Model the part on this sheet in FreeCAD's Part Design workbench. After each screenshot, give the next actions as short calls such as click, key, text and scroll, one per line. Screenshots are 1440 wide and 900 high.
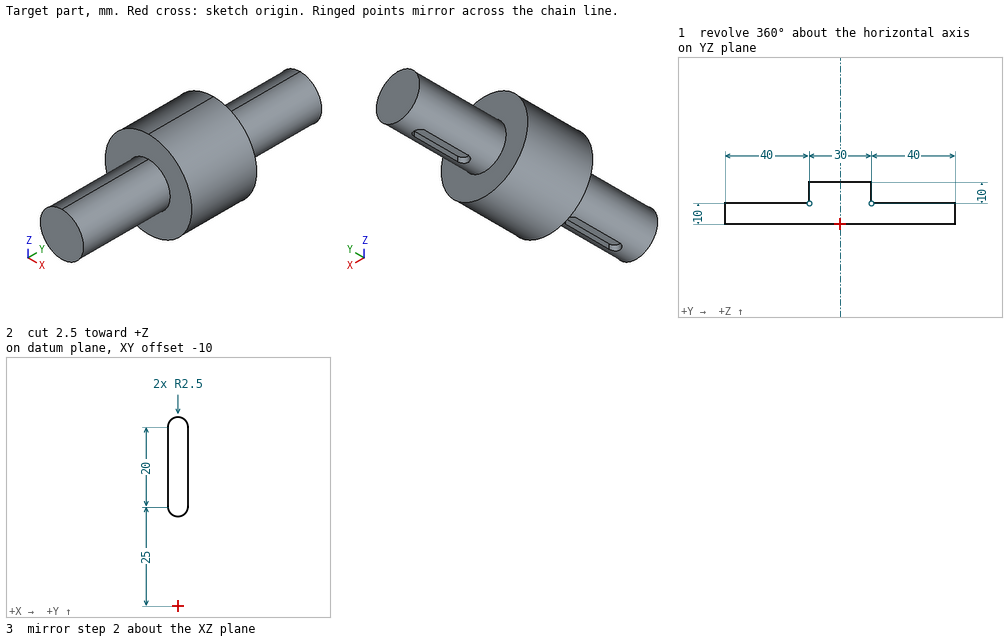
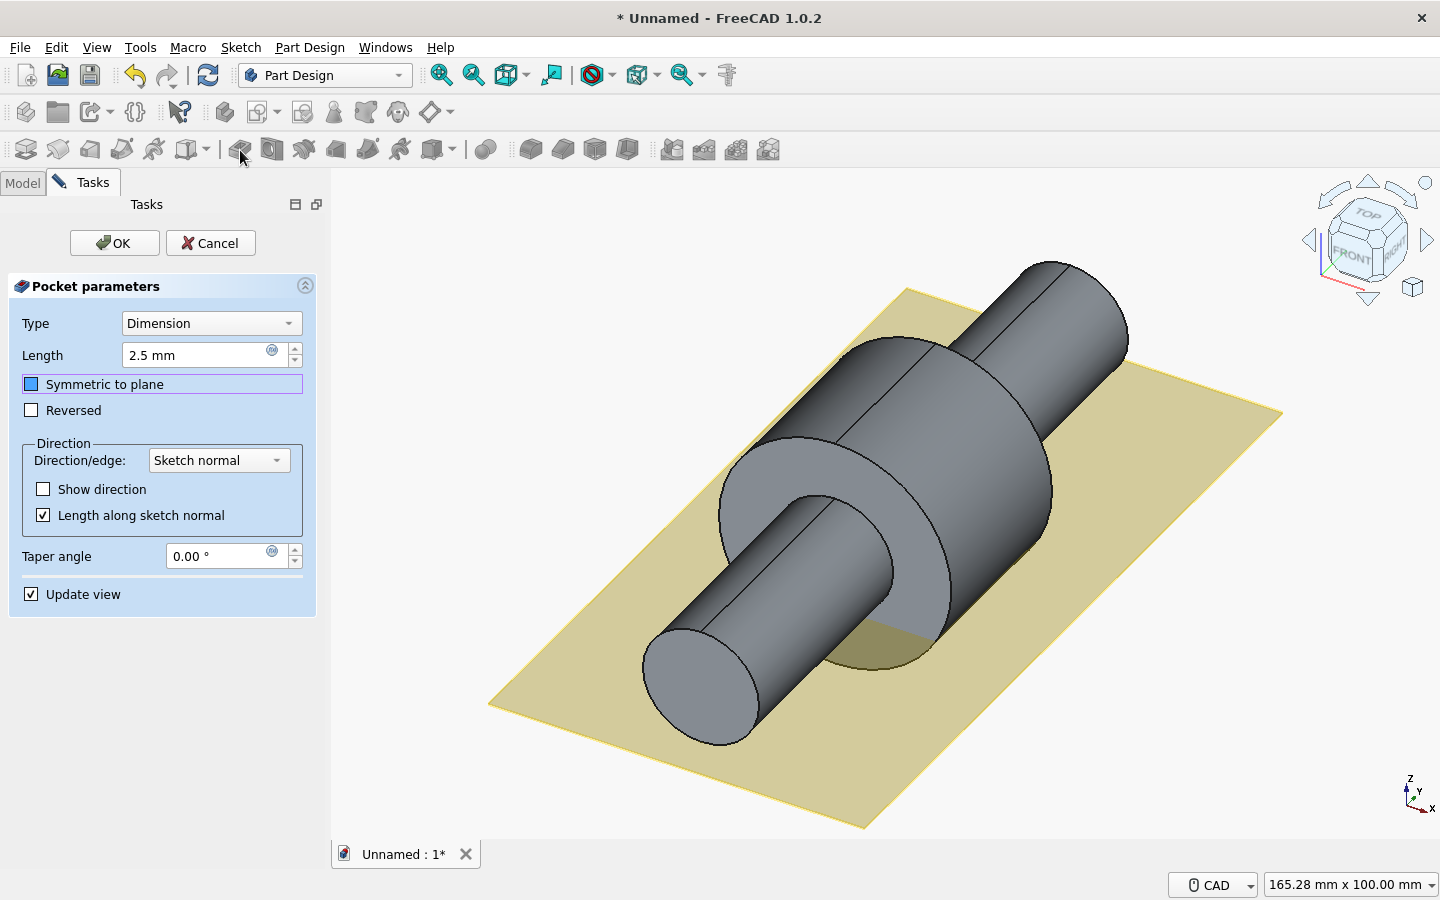
click(30, 410)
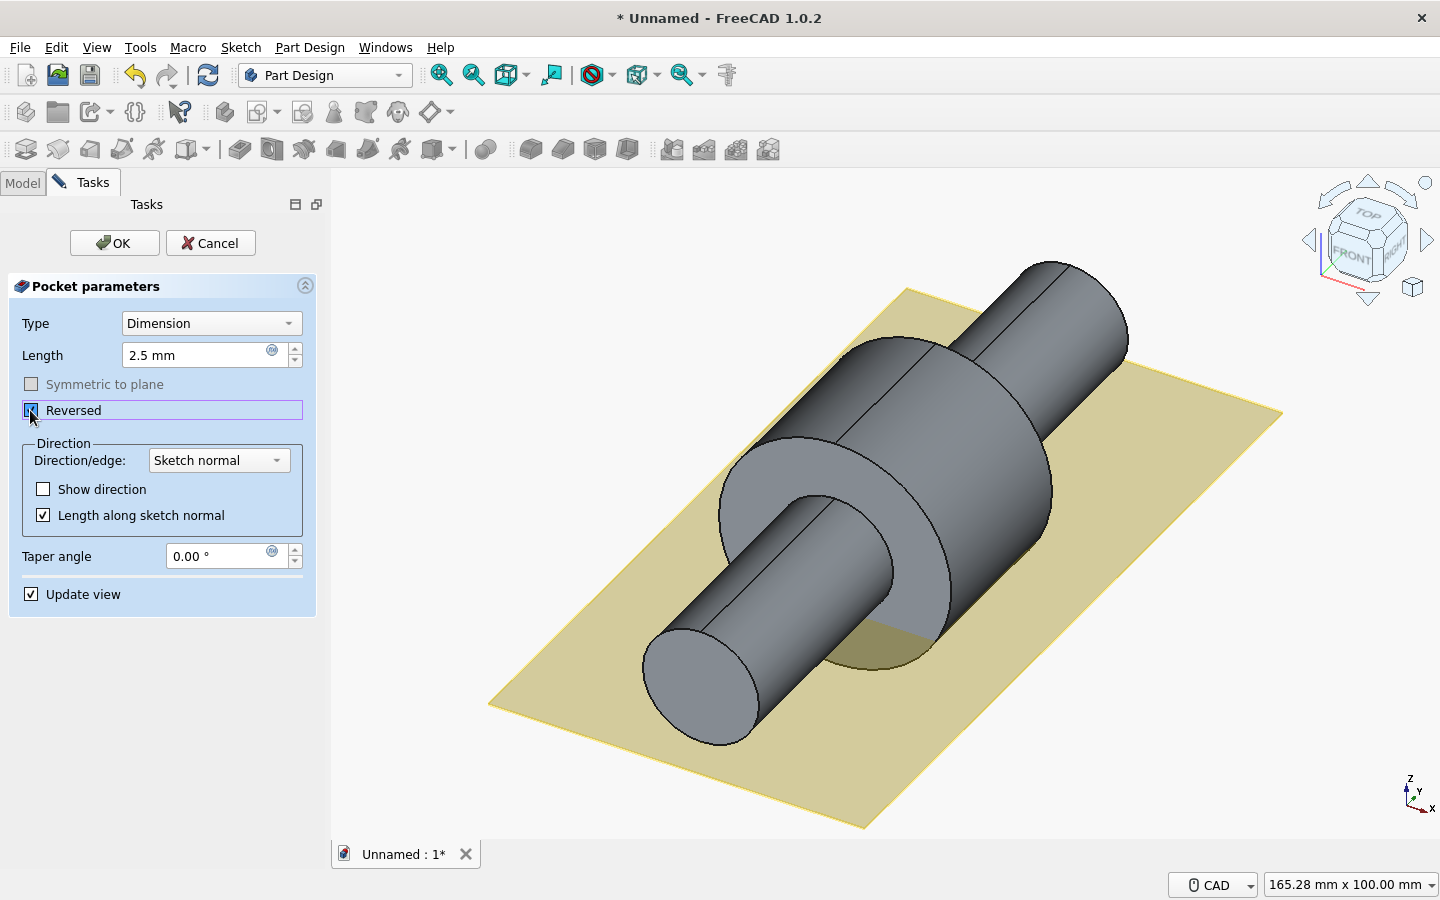
click(115, 243)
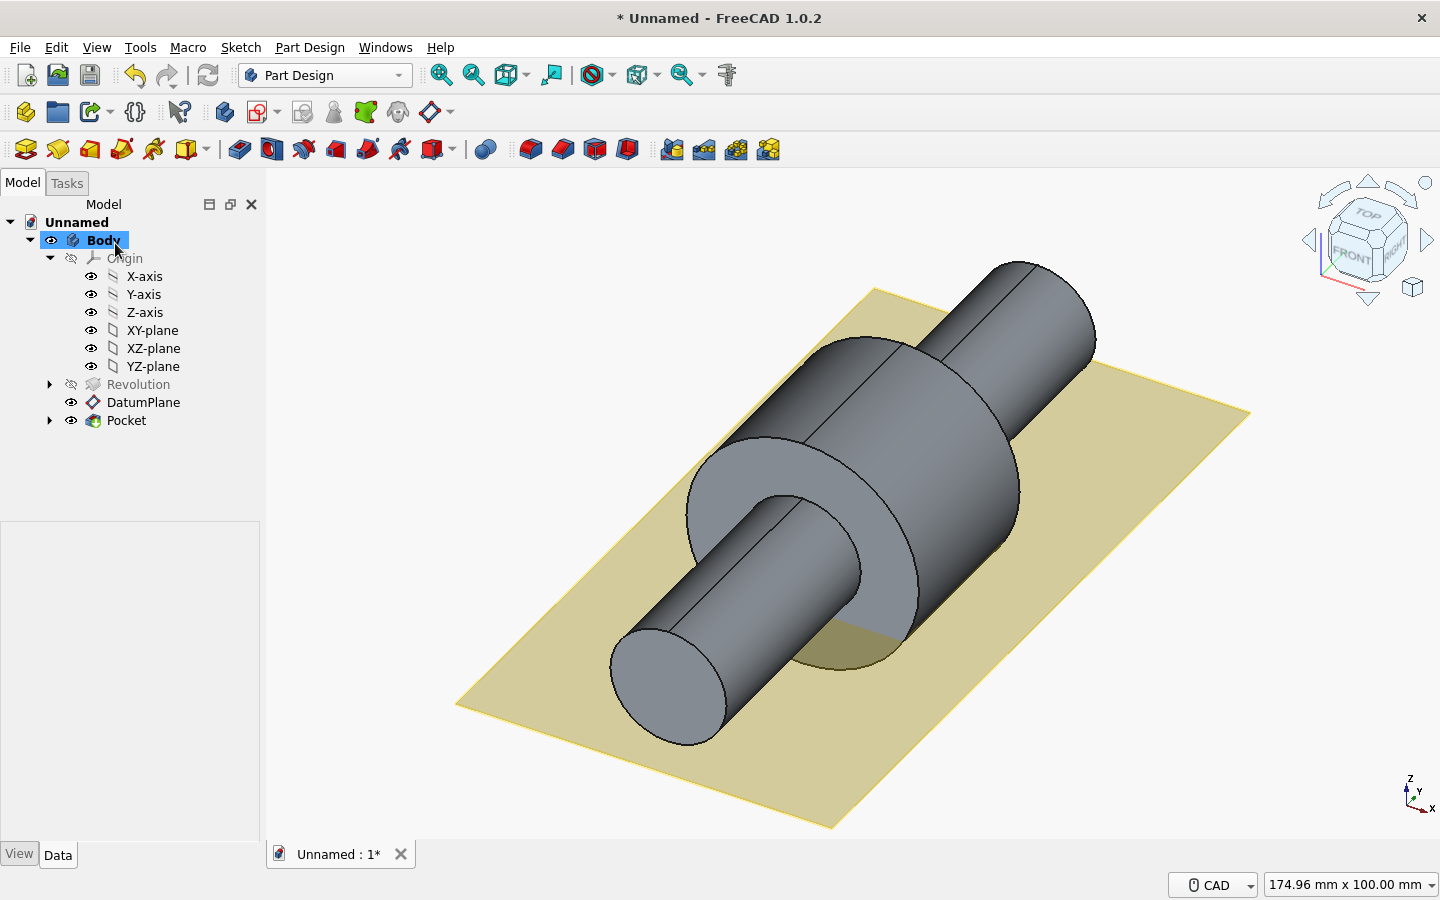
click(116, 402)
key(space)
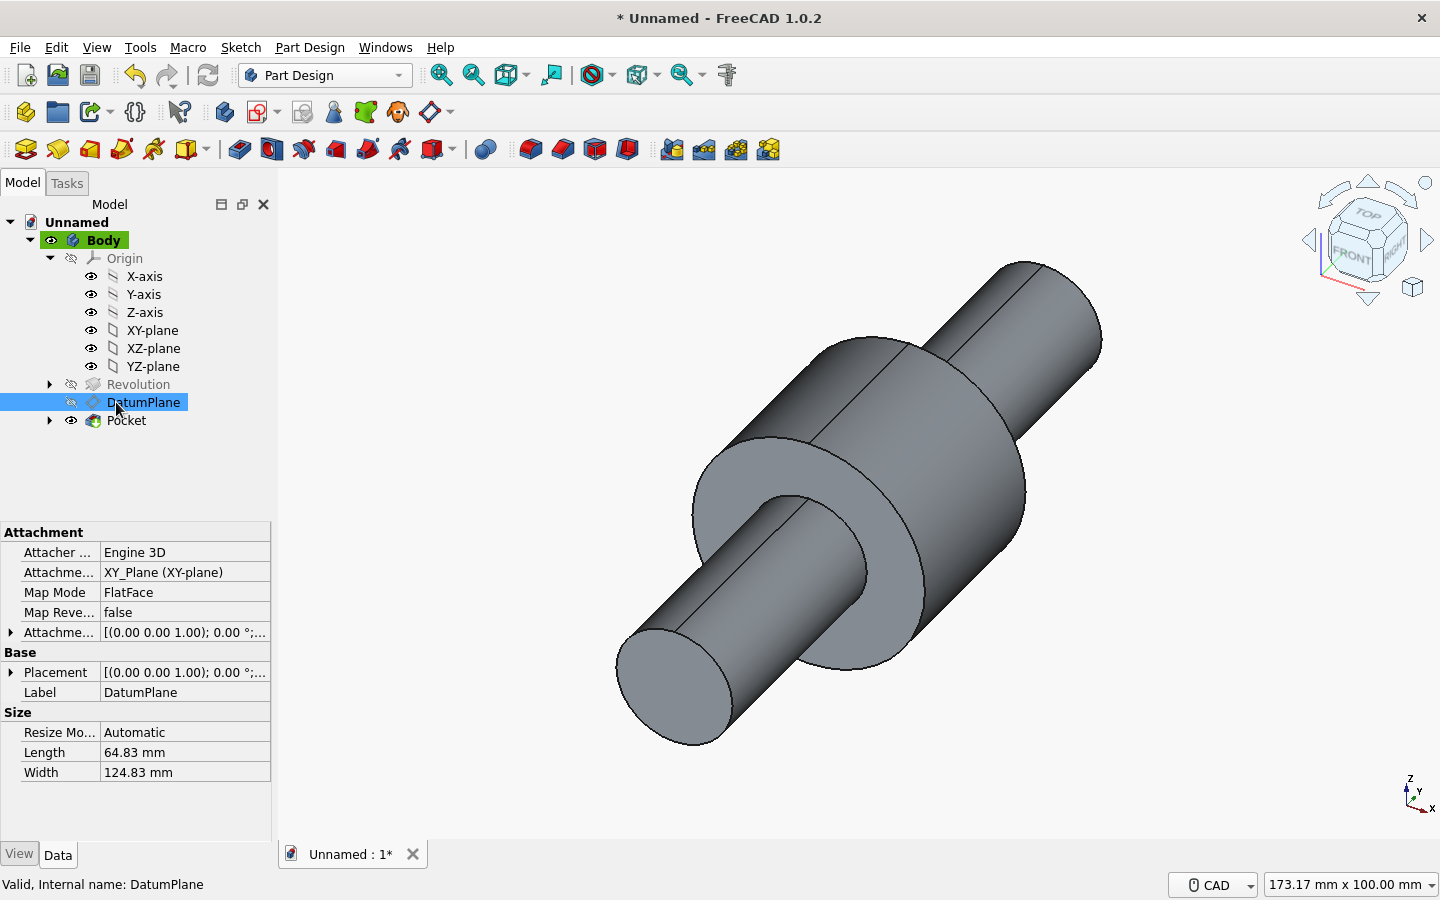
click(116, 420)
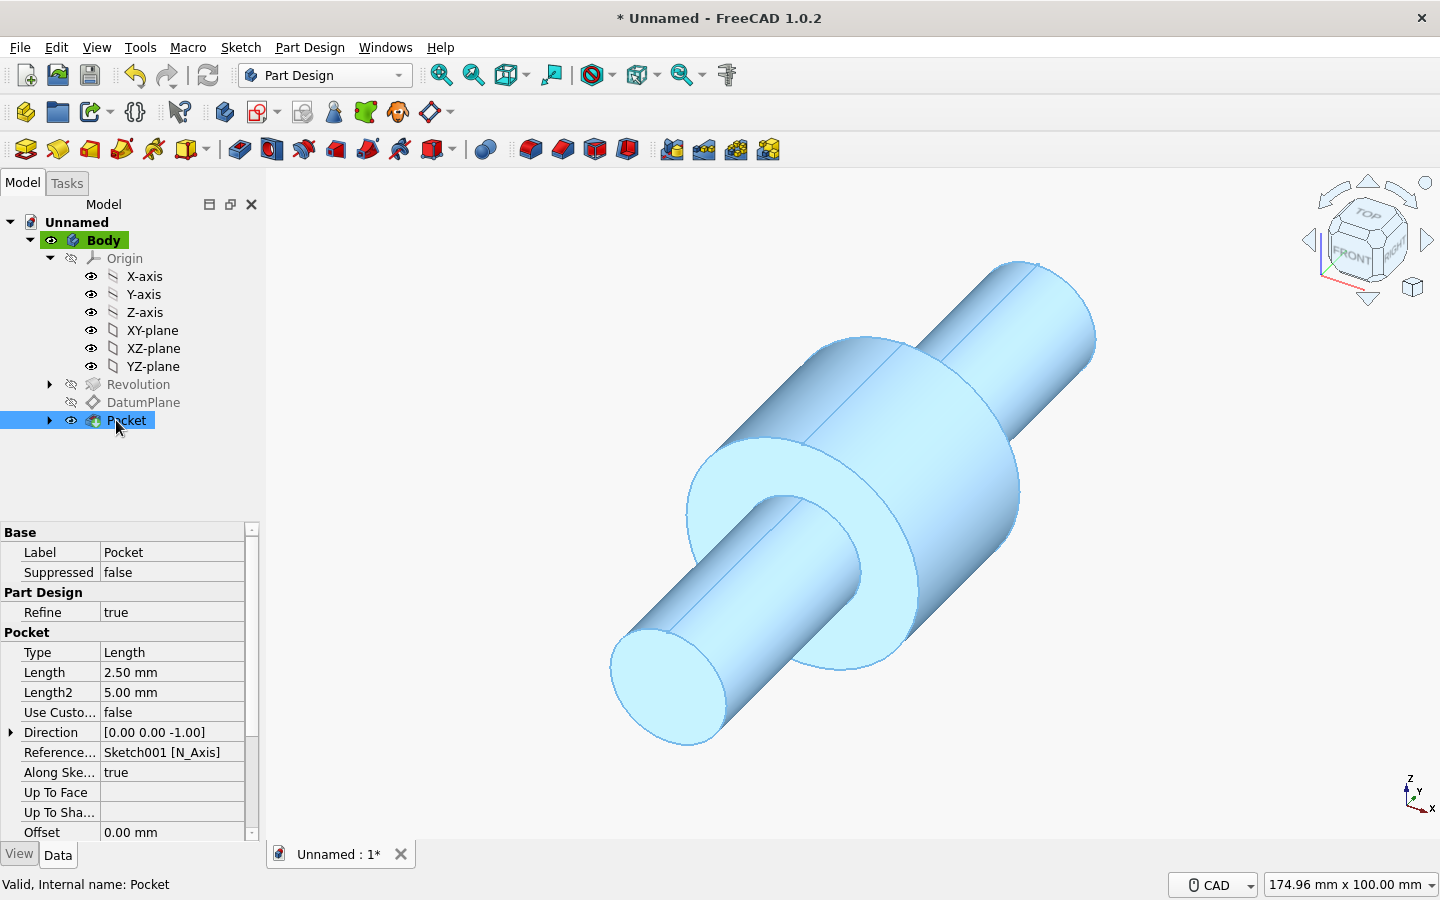
click(672, 150)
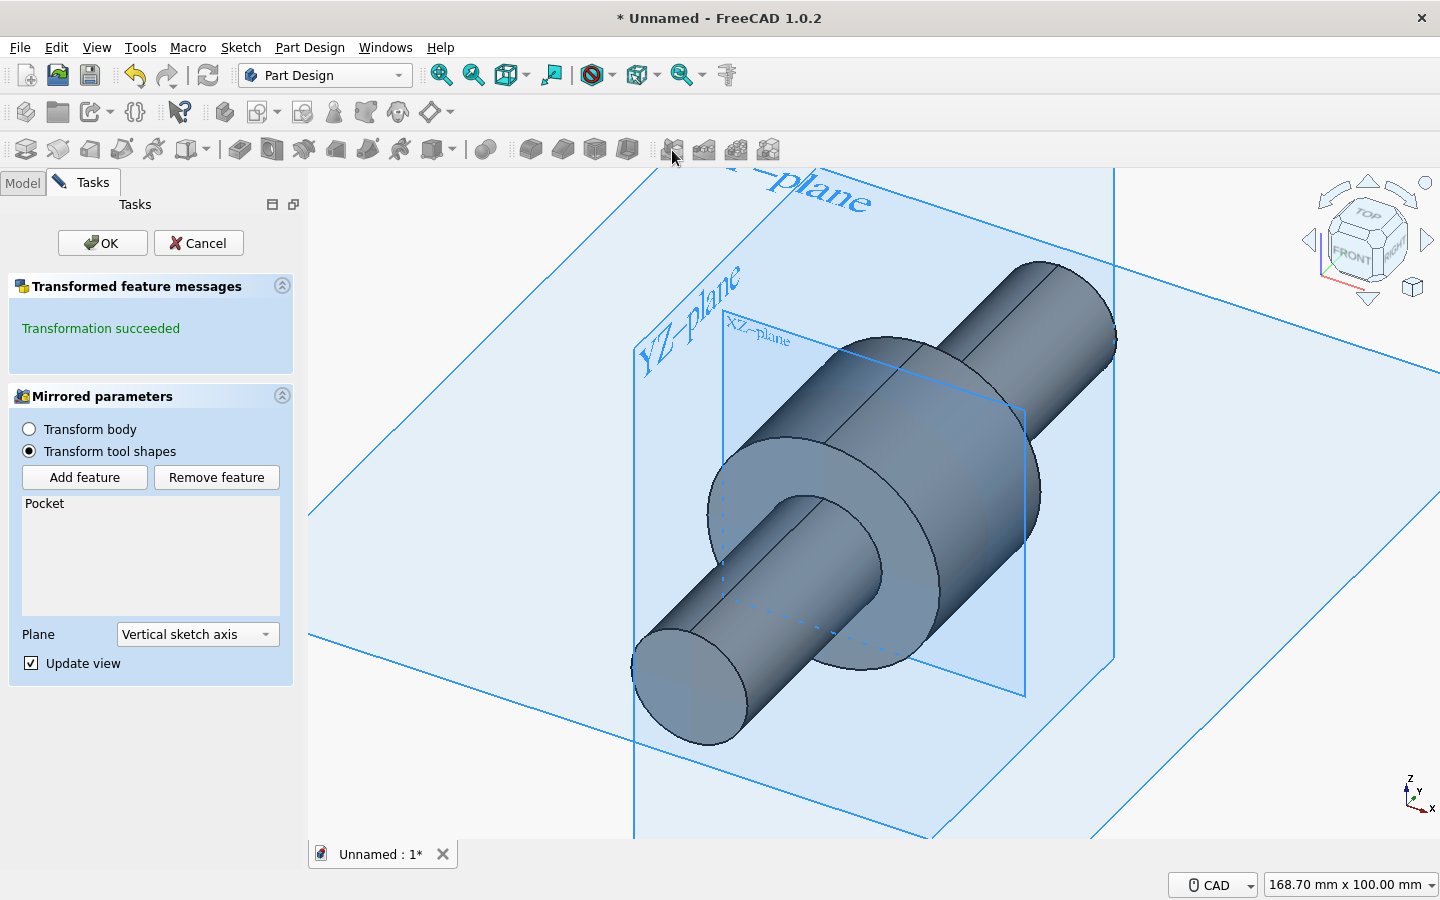
click(198, 634)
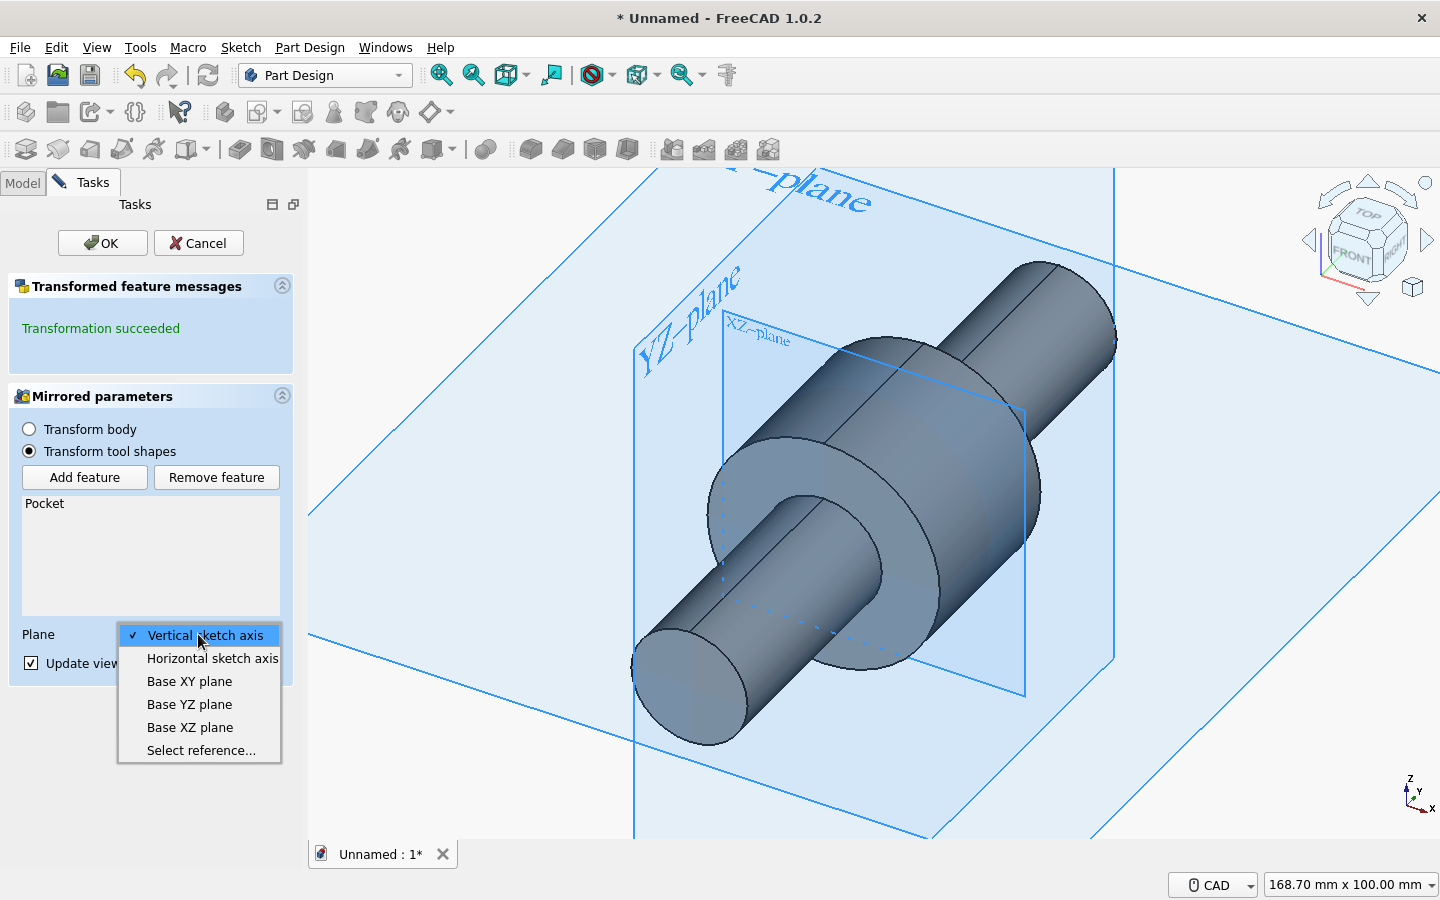
click(198, 728)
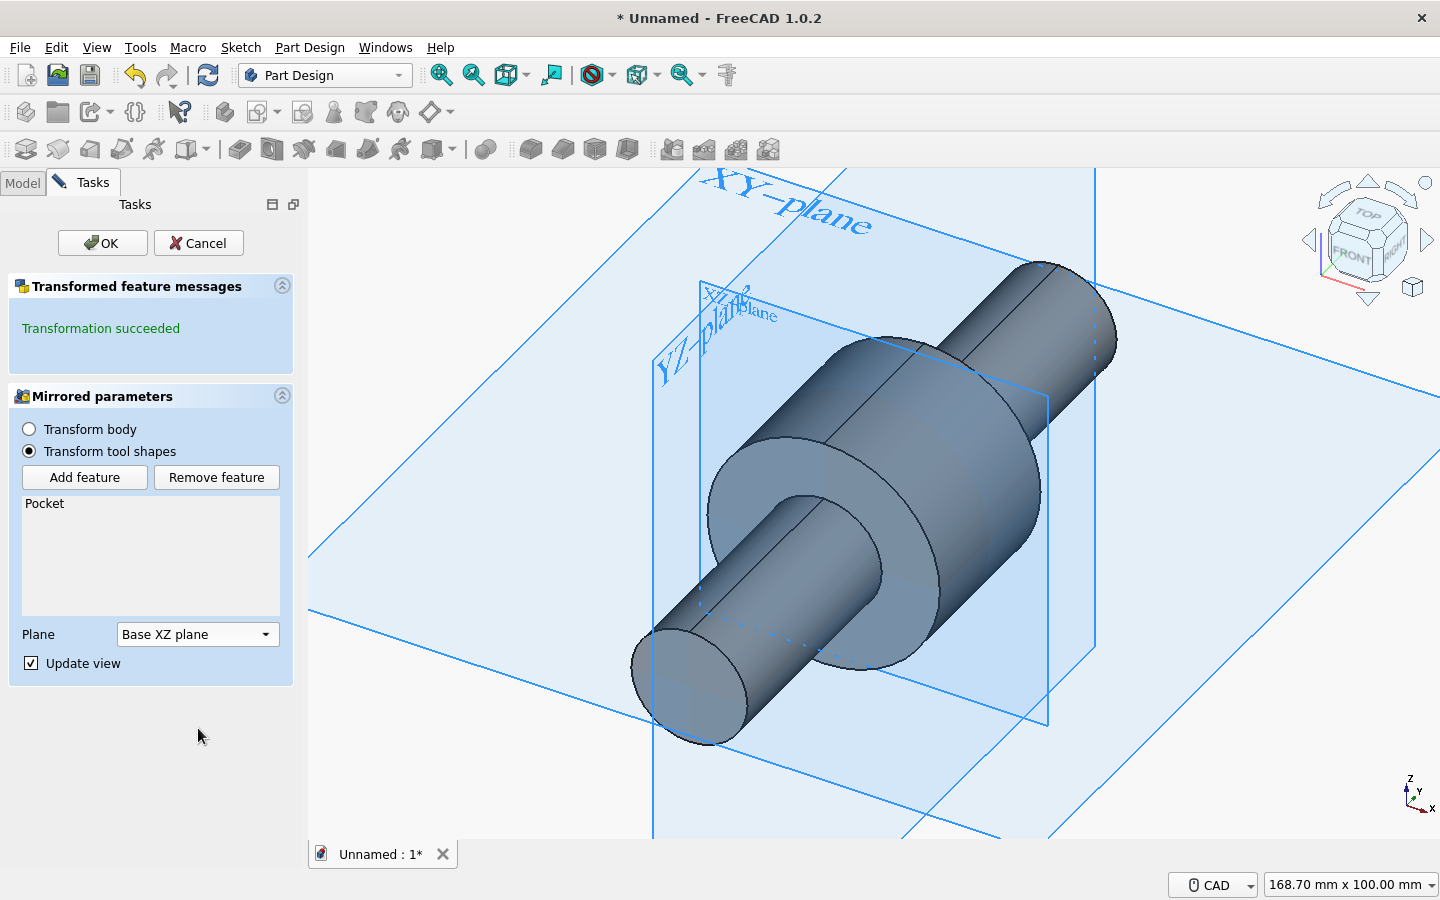
click(103, 243)